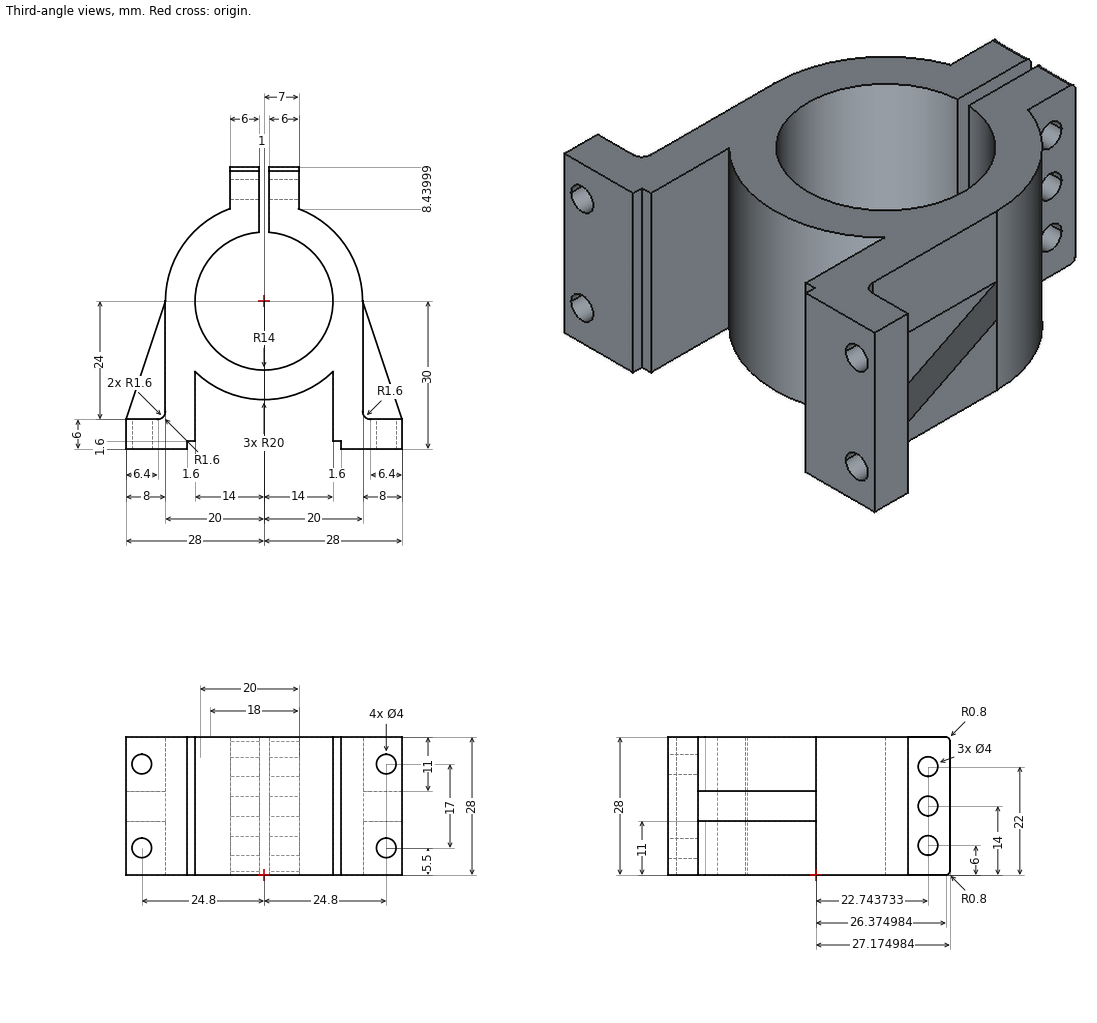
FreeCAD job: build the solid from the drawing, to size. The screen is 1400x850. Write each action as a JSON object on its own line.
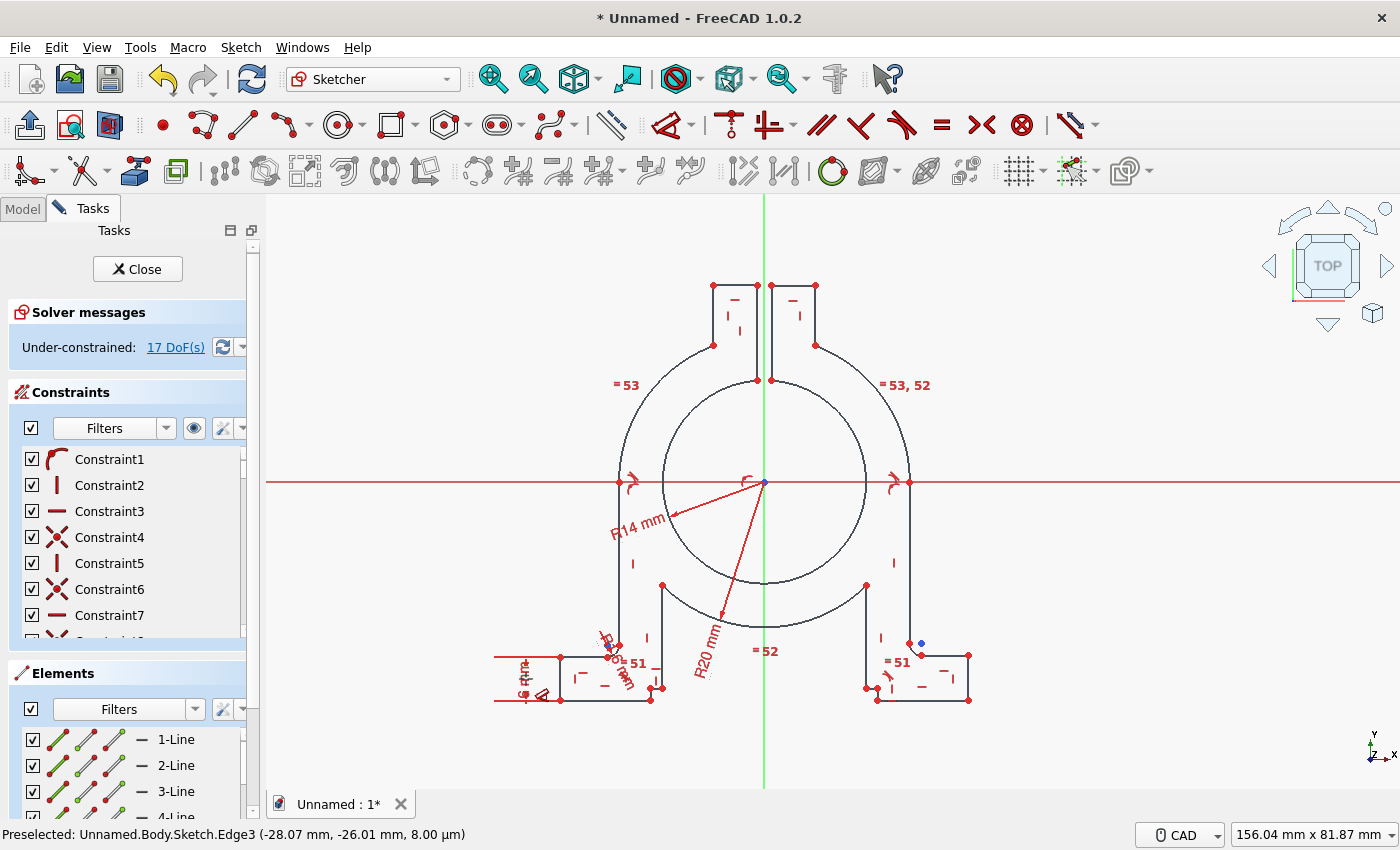
{"action": "left_click", "coordinate": [968, 687]}
{"action": "left_click", "coordinate": [1002, 678]}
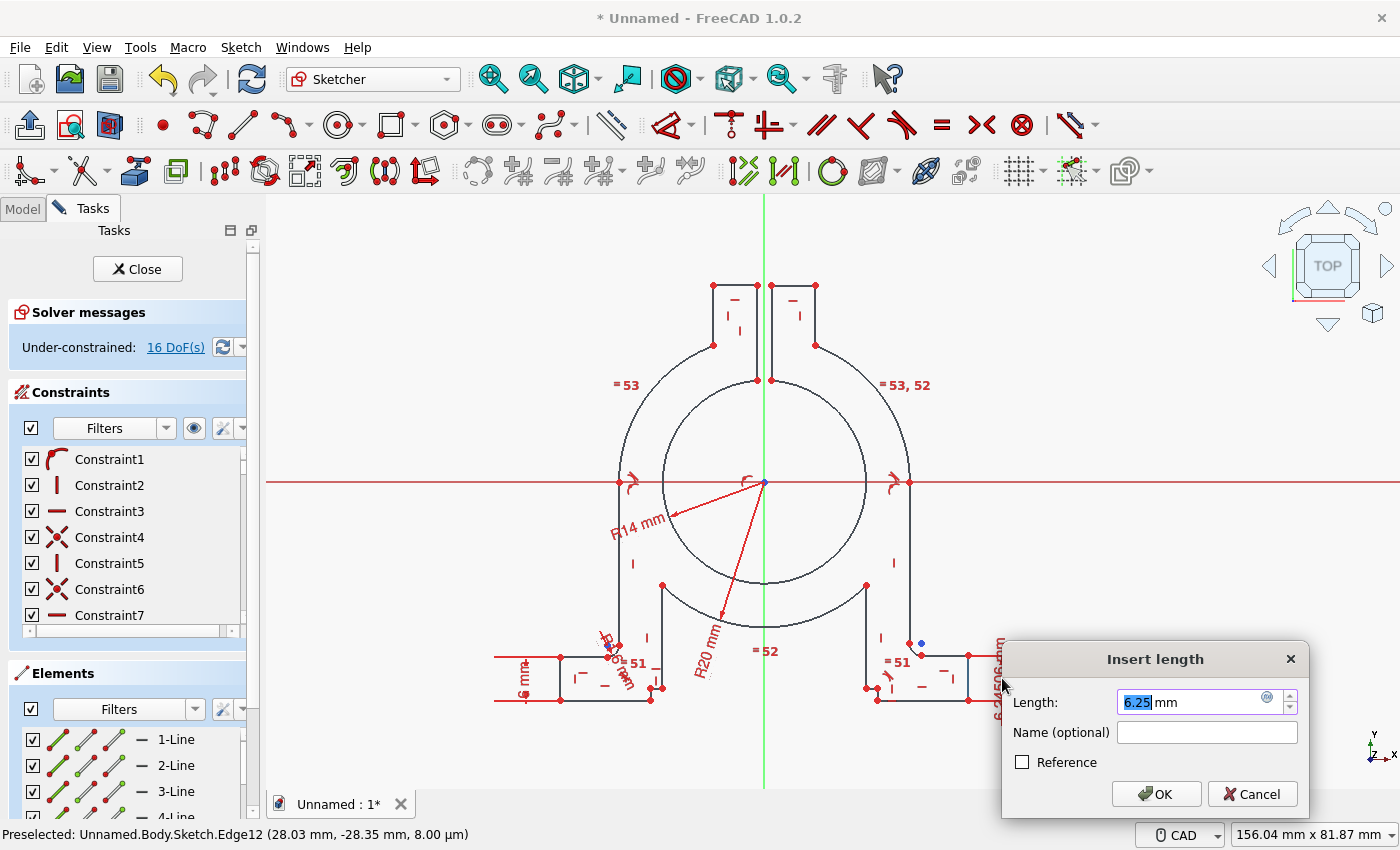
{"action": "type", "text": "6"}
{"action": "key", "text": "Return"}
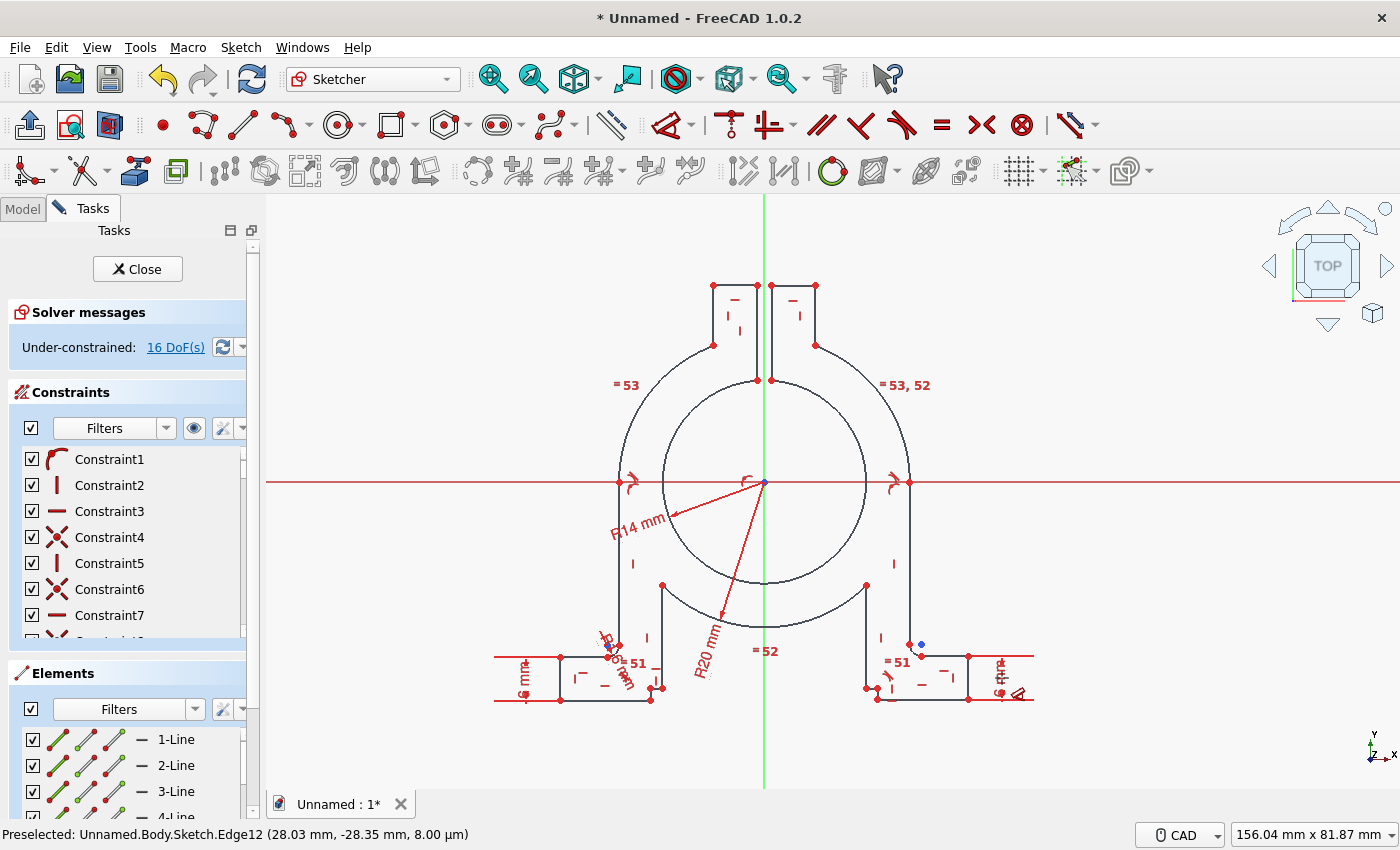
{"action": "left_click", "coordinate": [802, 286]}
{"action": "left_click", "coordinate": [793, 252]}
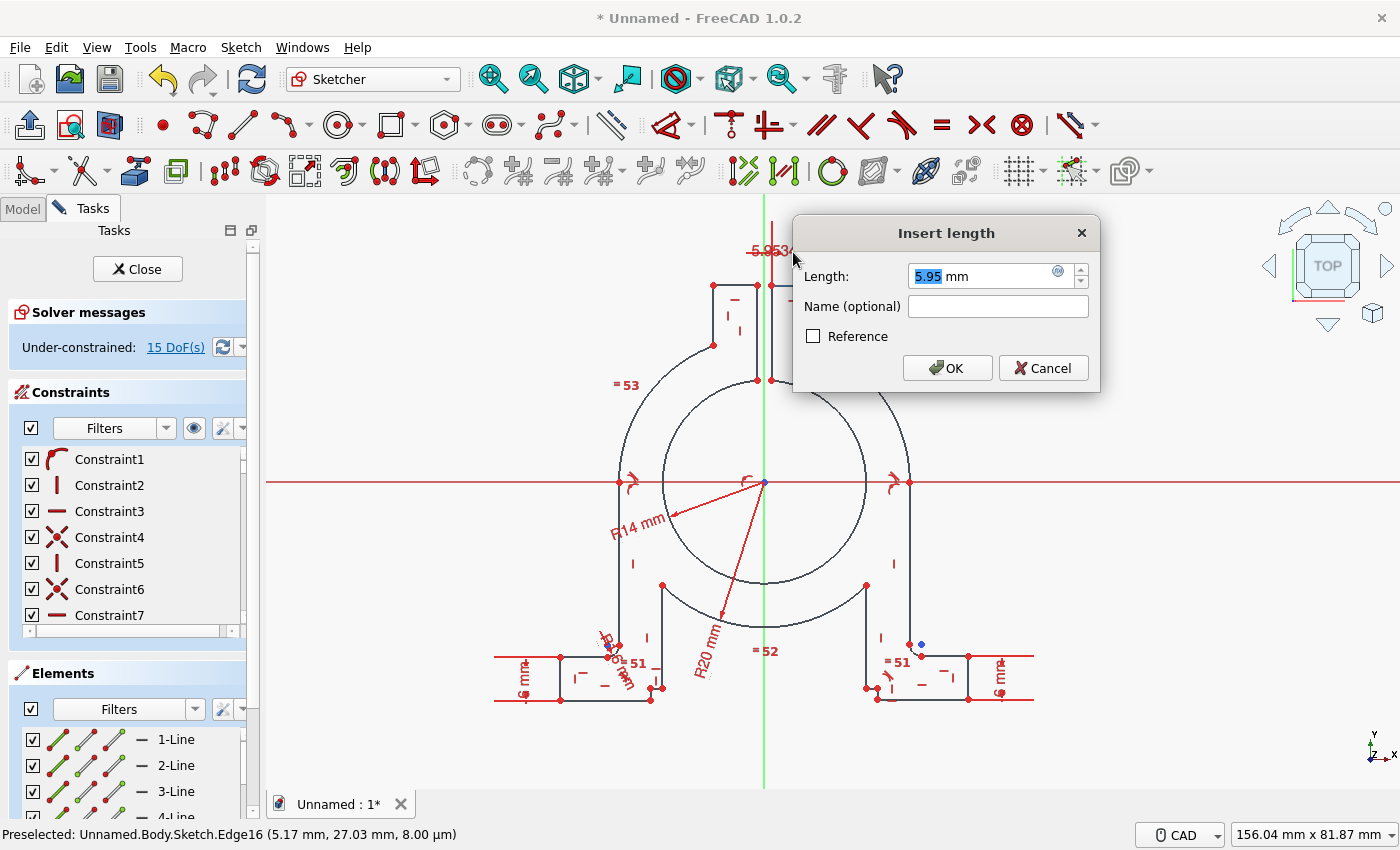
{"action": "type", "text": "6"}
{"action": "key", "text": "Return"}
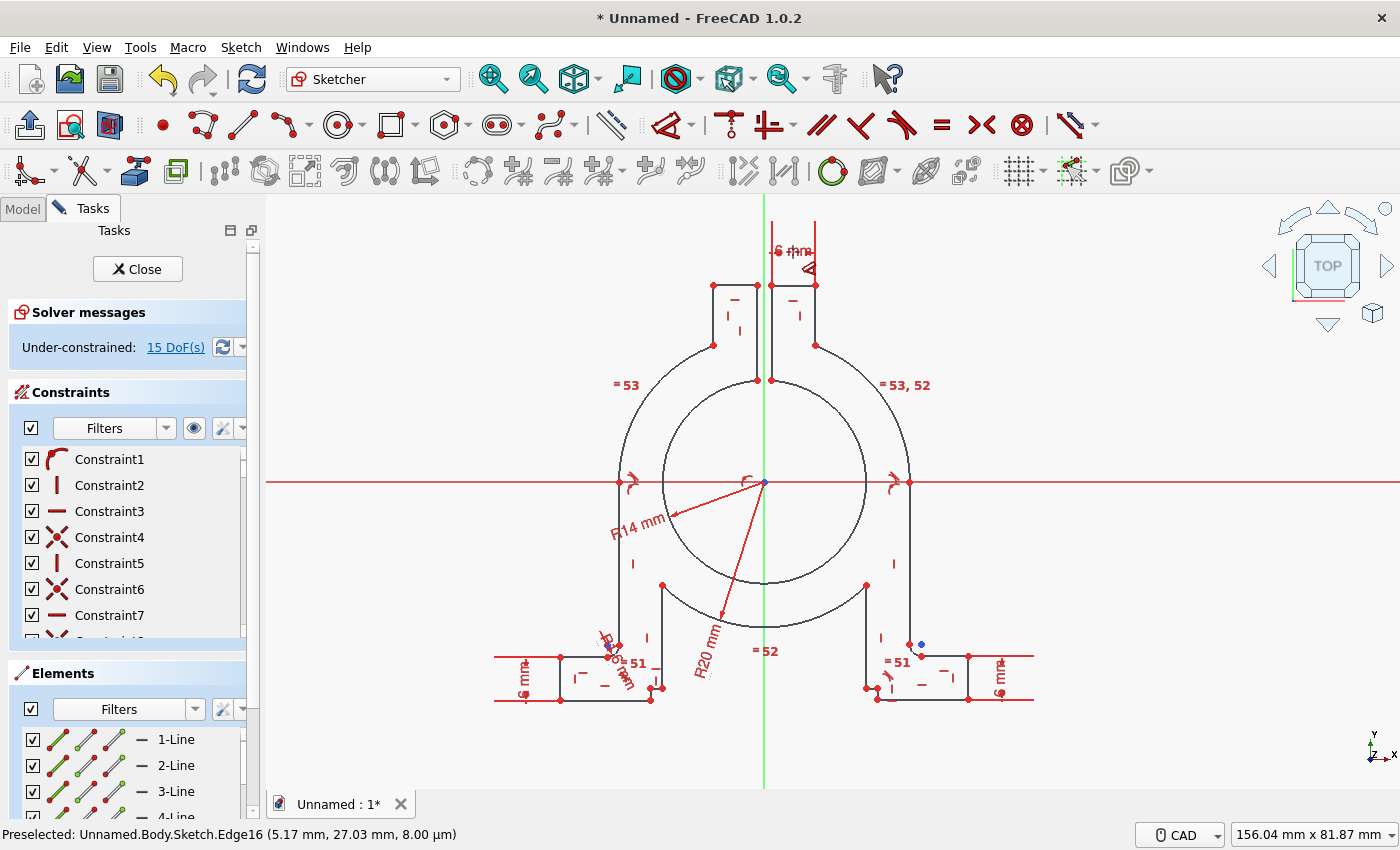
{"action": "left_click", "coordinate": [744, 285]}
{"action": "left_click", "coordinate": [720, 251]}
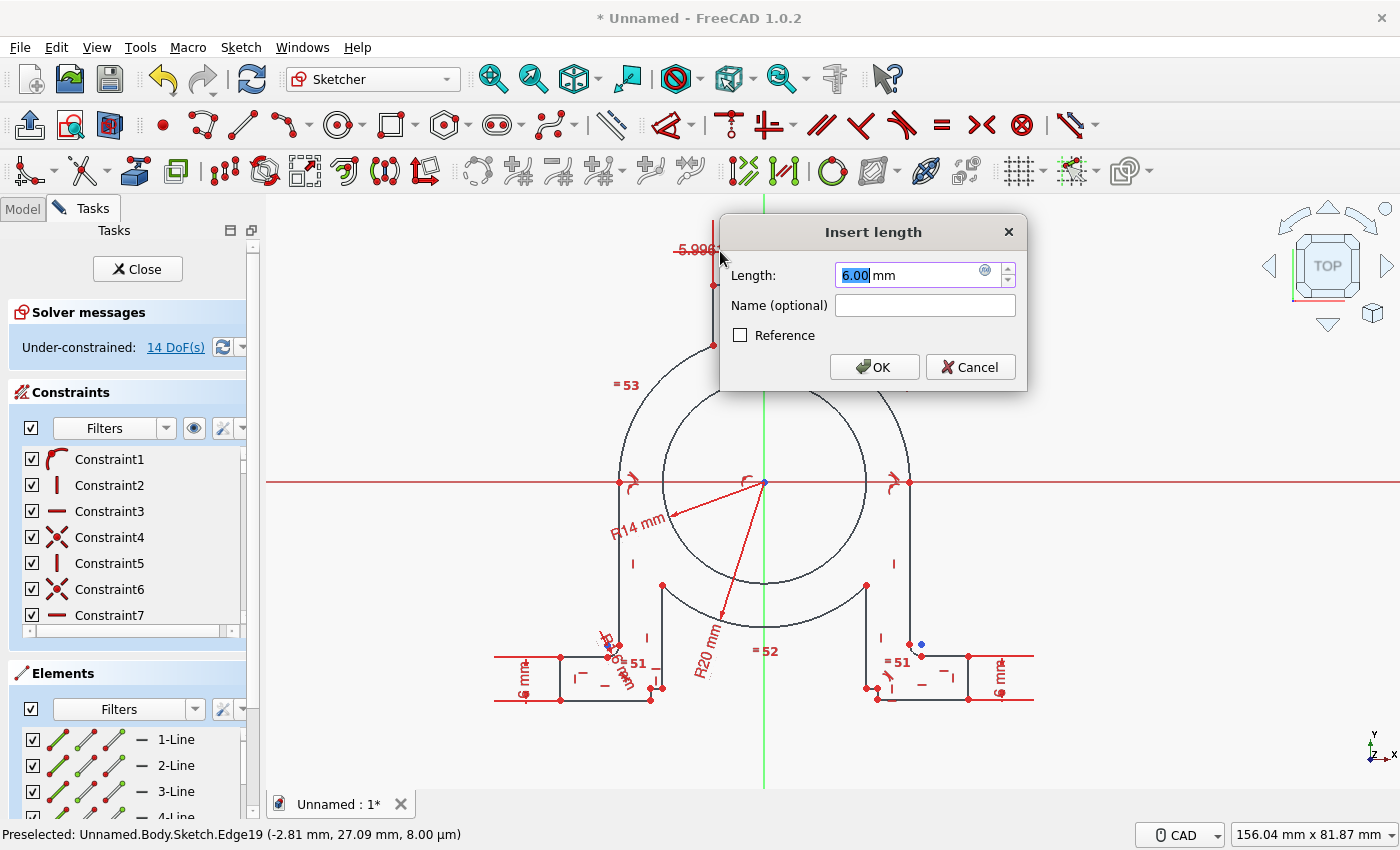
{"action": "type", "text": "6"}
{"action": "key", "text": "Return"}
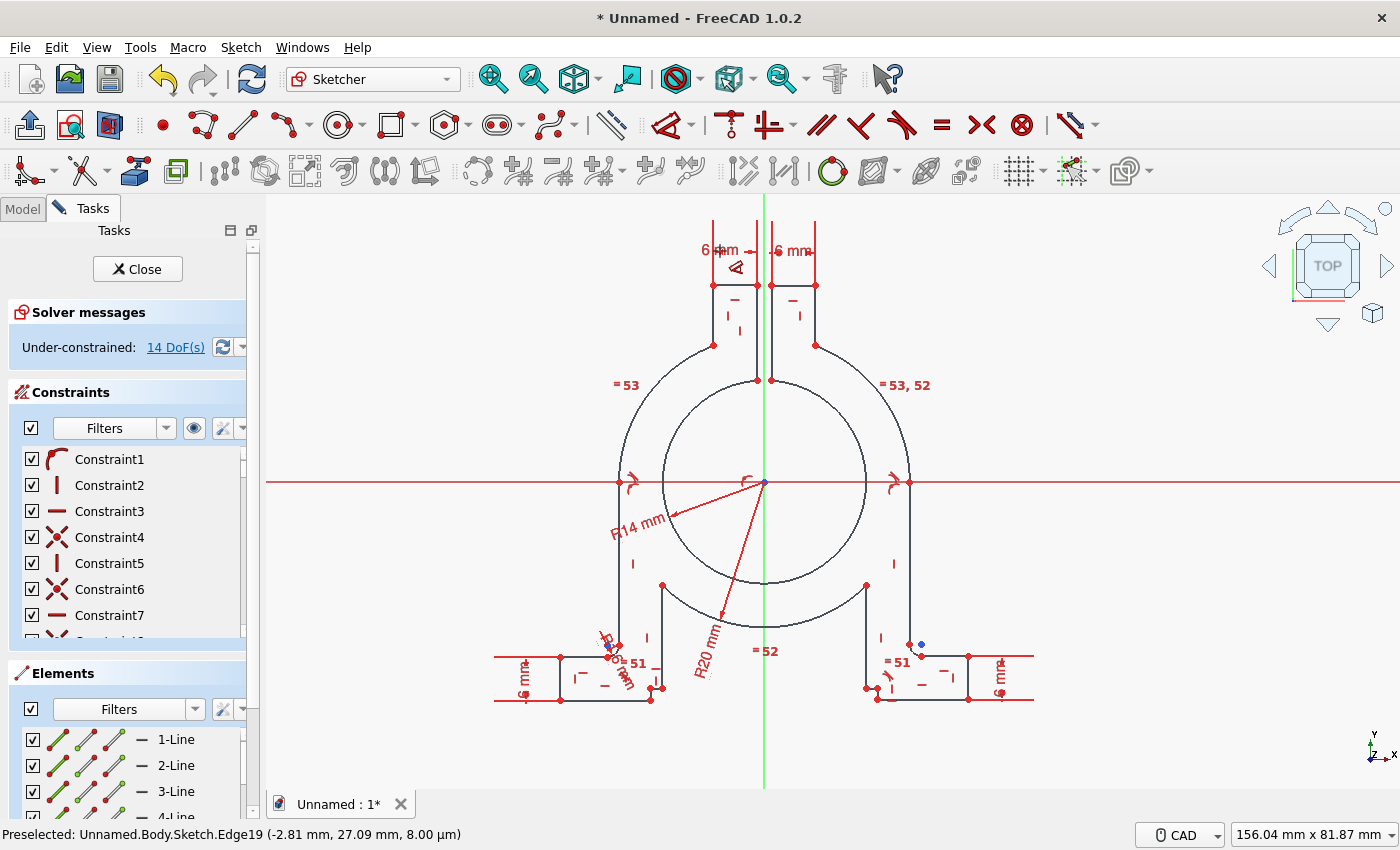
{"action": "left_click", "coordinate": [815, 346]}
{"action": "left_click", "coordinate": [790, 312]}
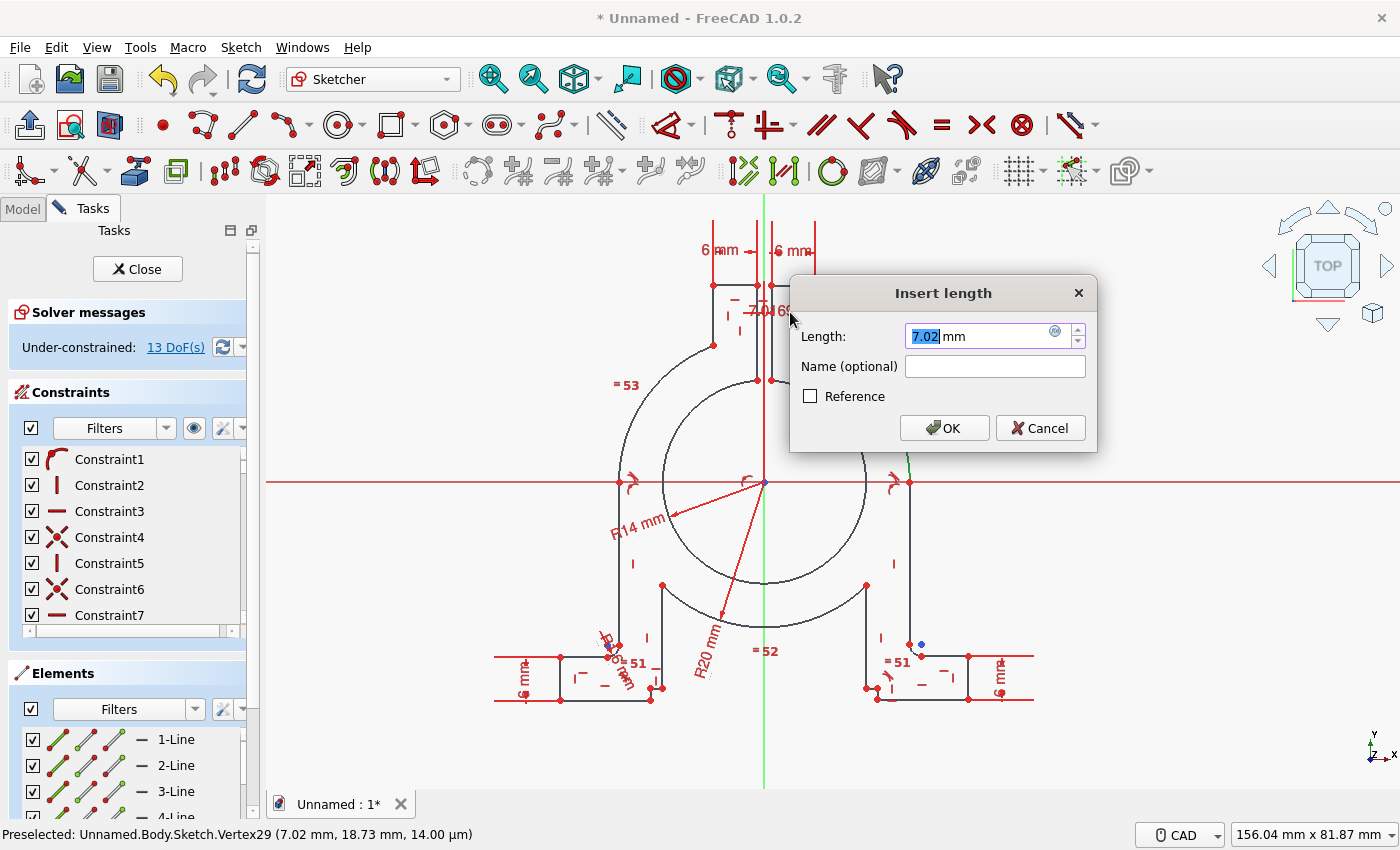
{"action": "type", "text": "7"}
{"action": "key", "text": "Return"}